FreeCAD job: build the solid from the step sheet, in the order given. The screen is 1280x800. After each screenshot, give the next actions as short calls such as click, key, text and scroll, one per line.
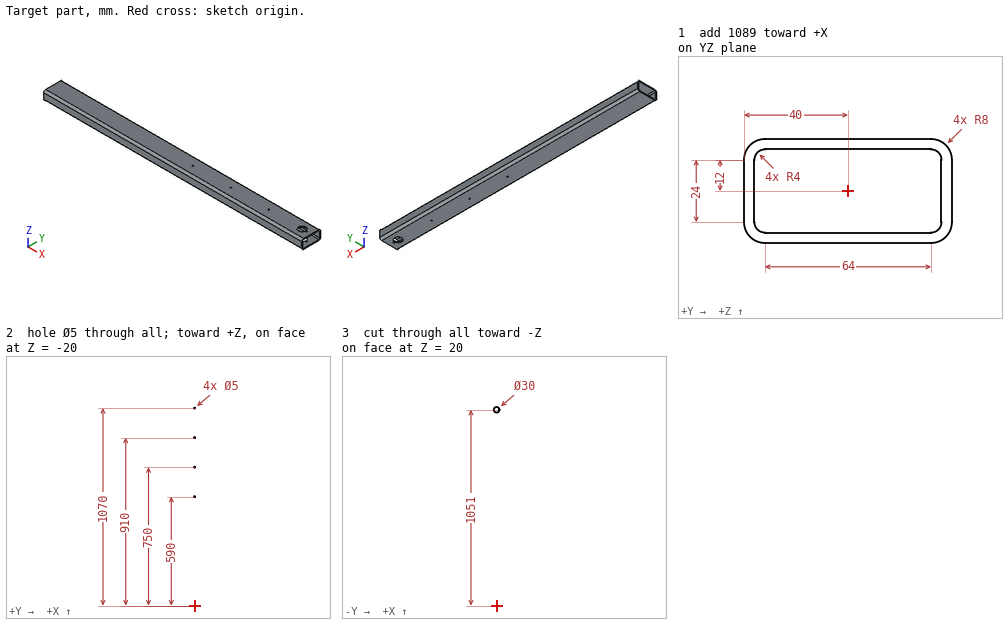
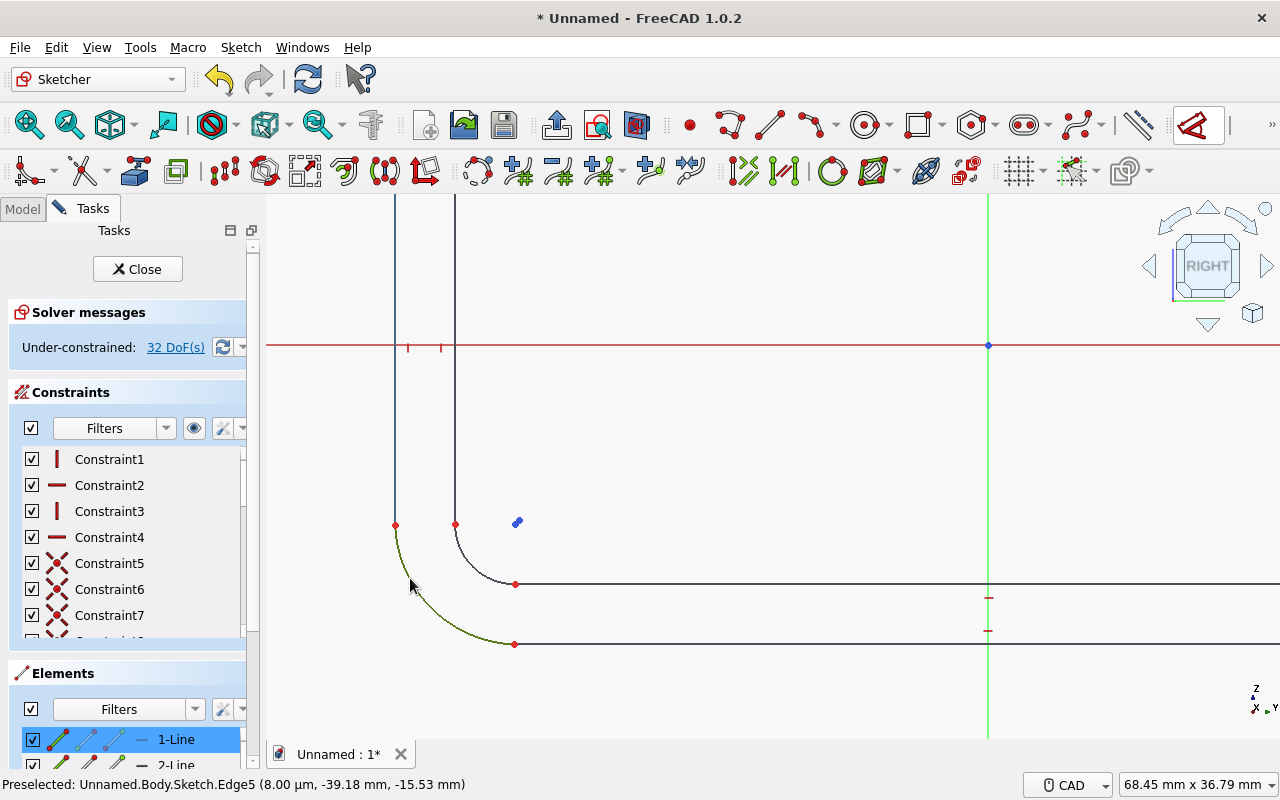
key(t)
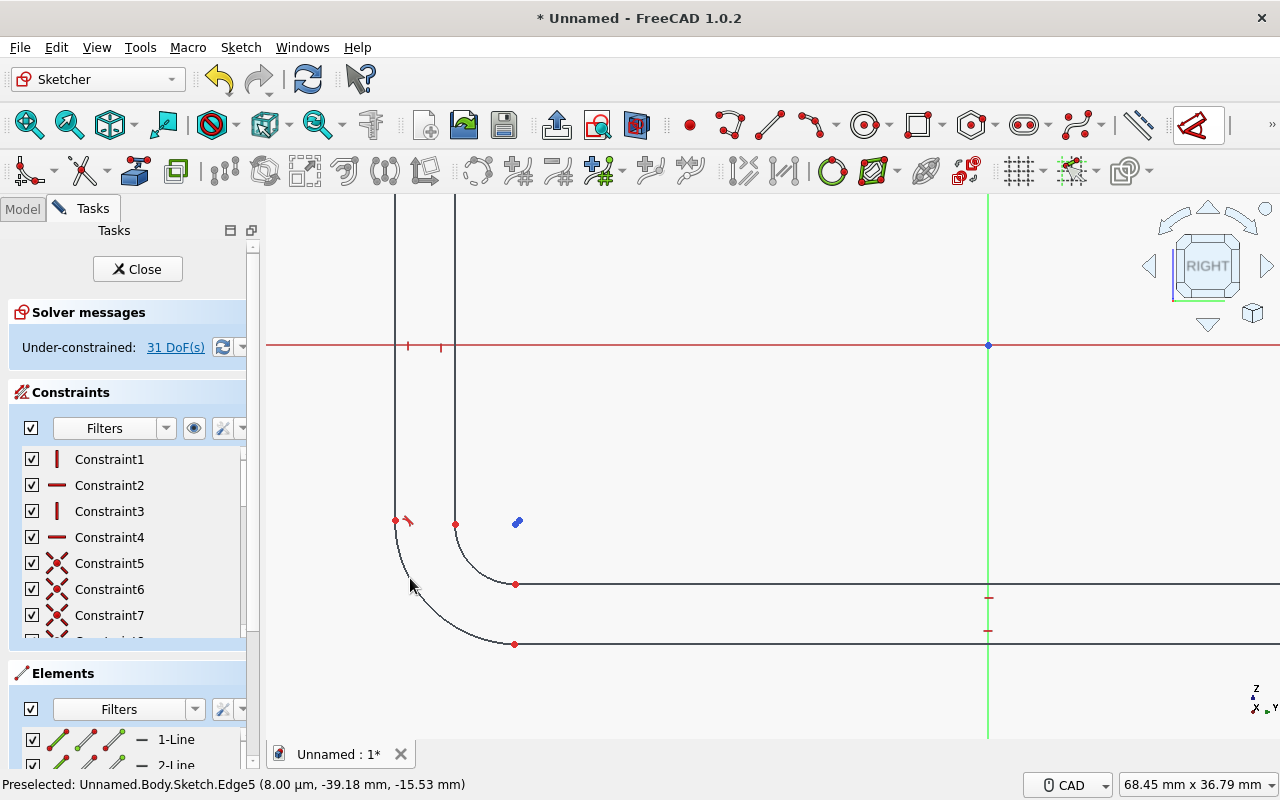
click(395, 275)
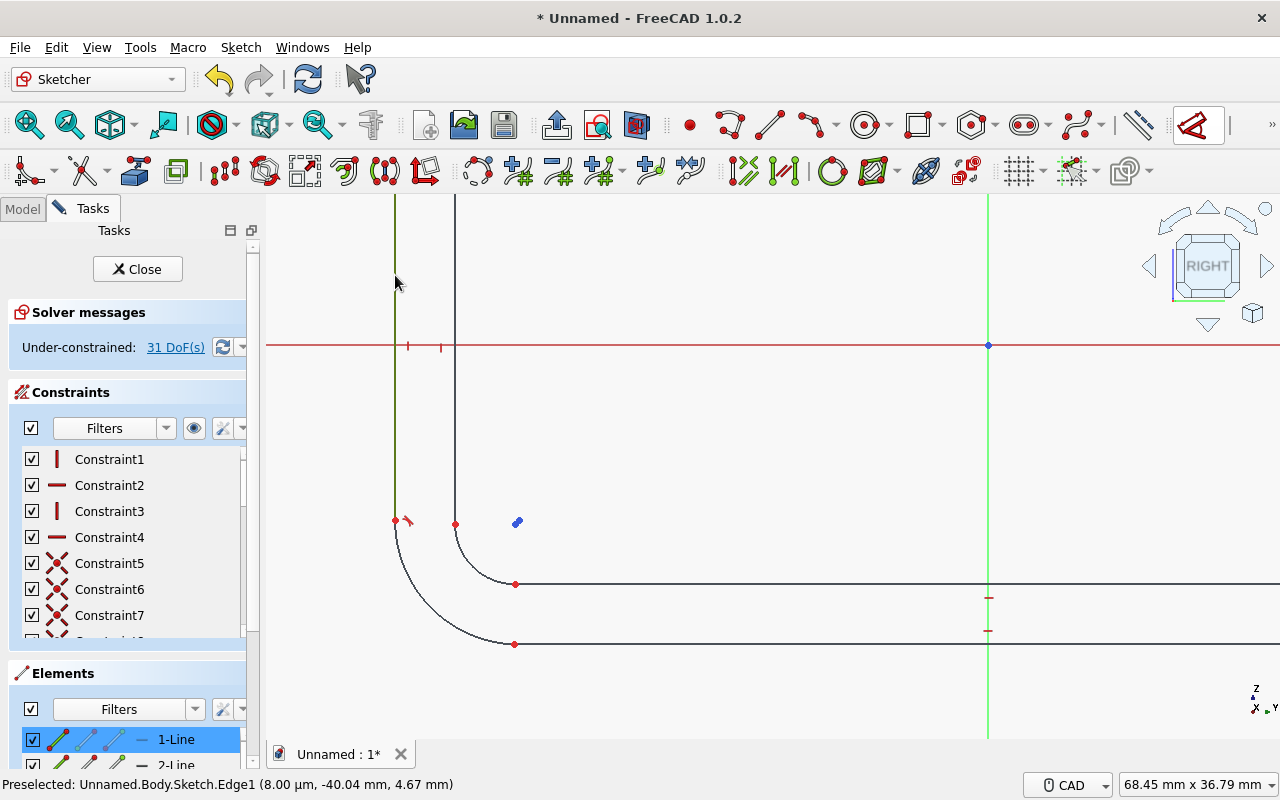
scroll(473, 566, down, 4)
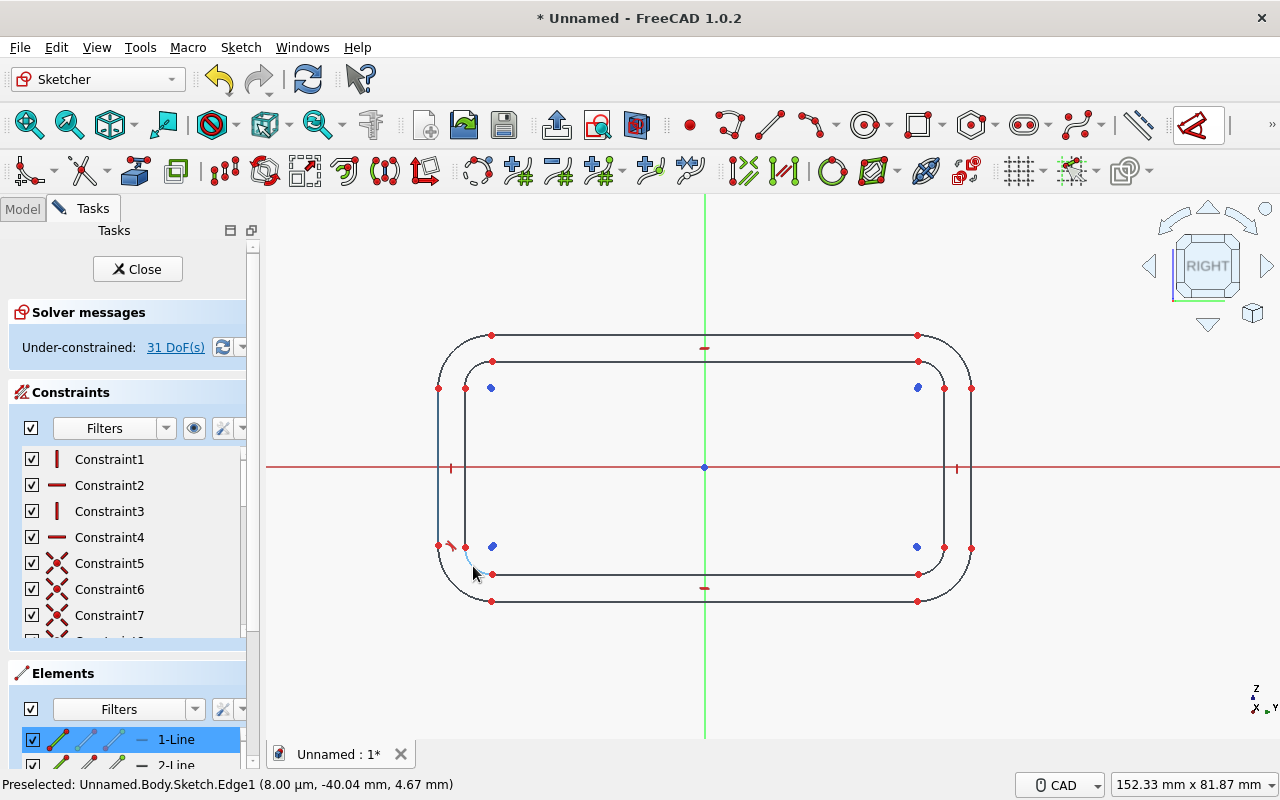
click(467, 341)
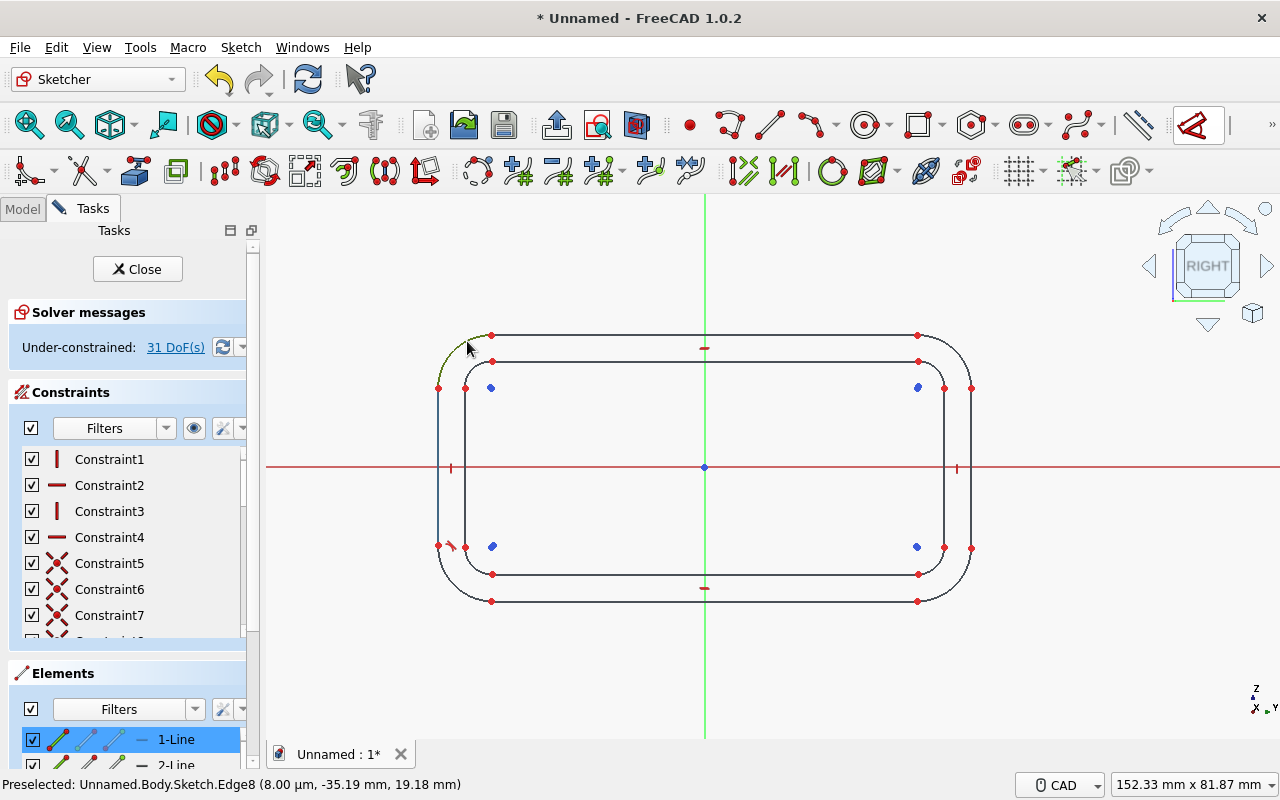
key(t)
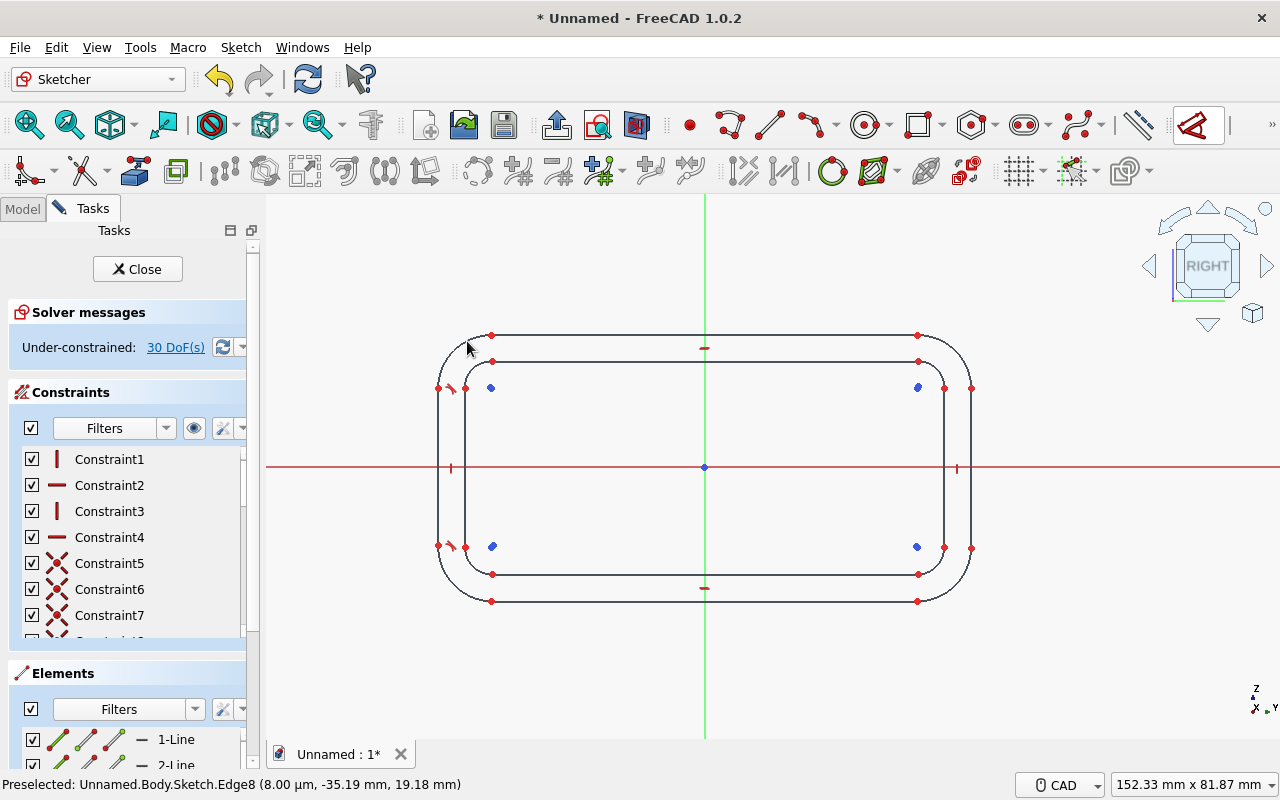
click(619, 602)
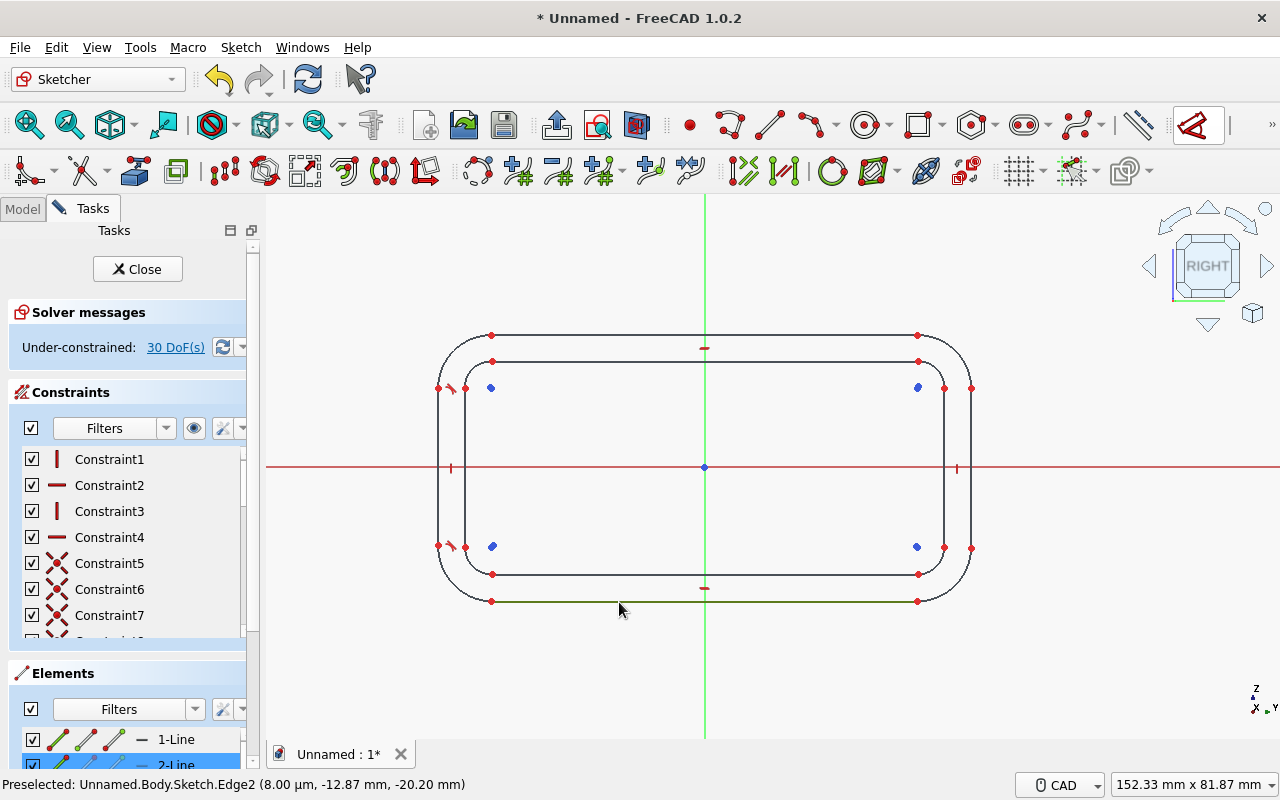
click(444, 571)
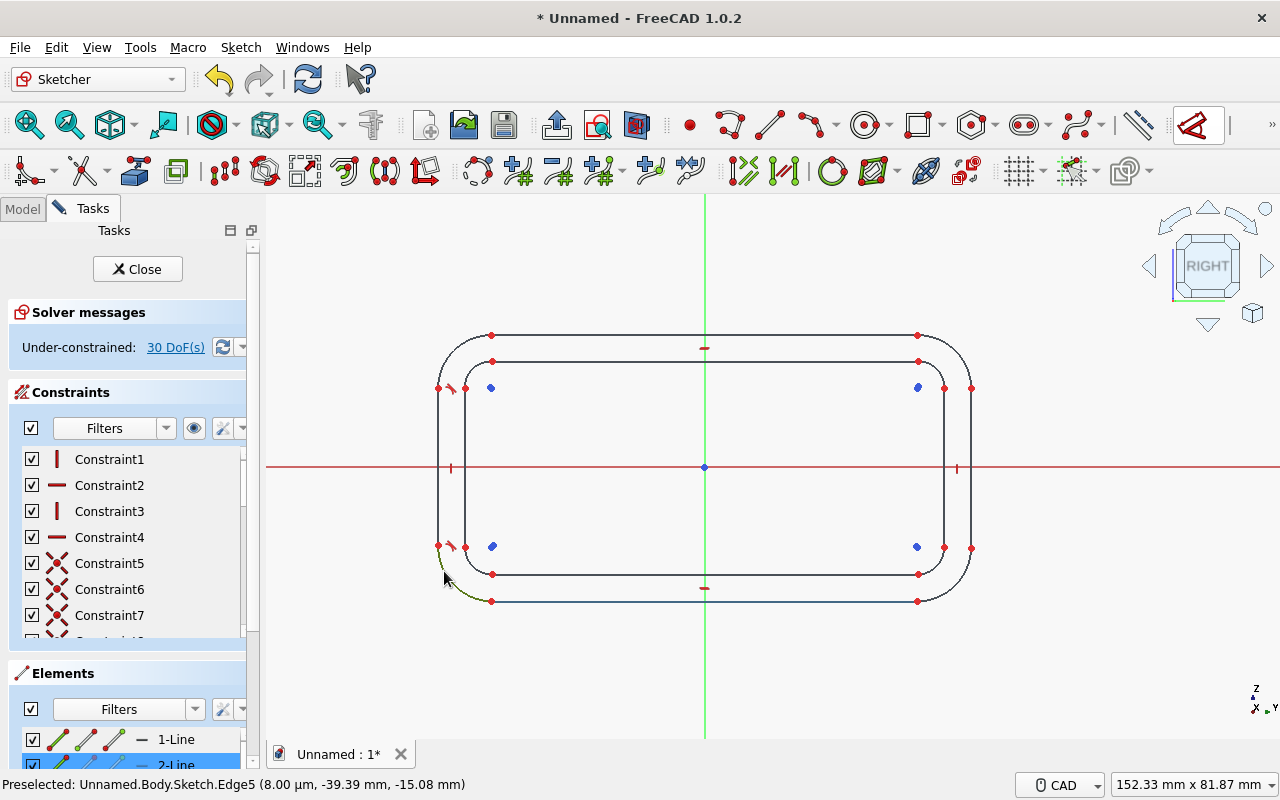
key(t)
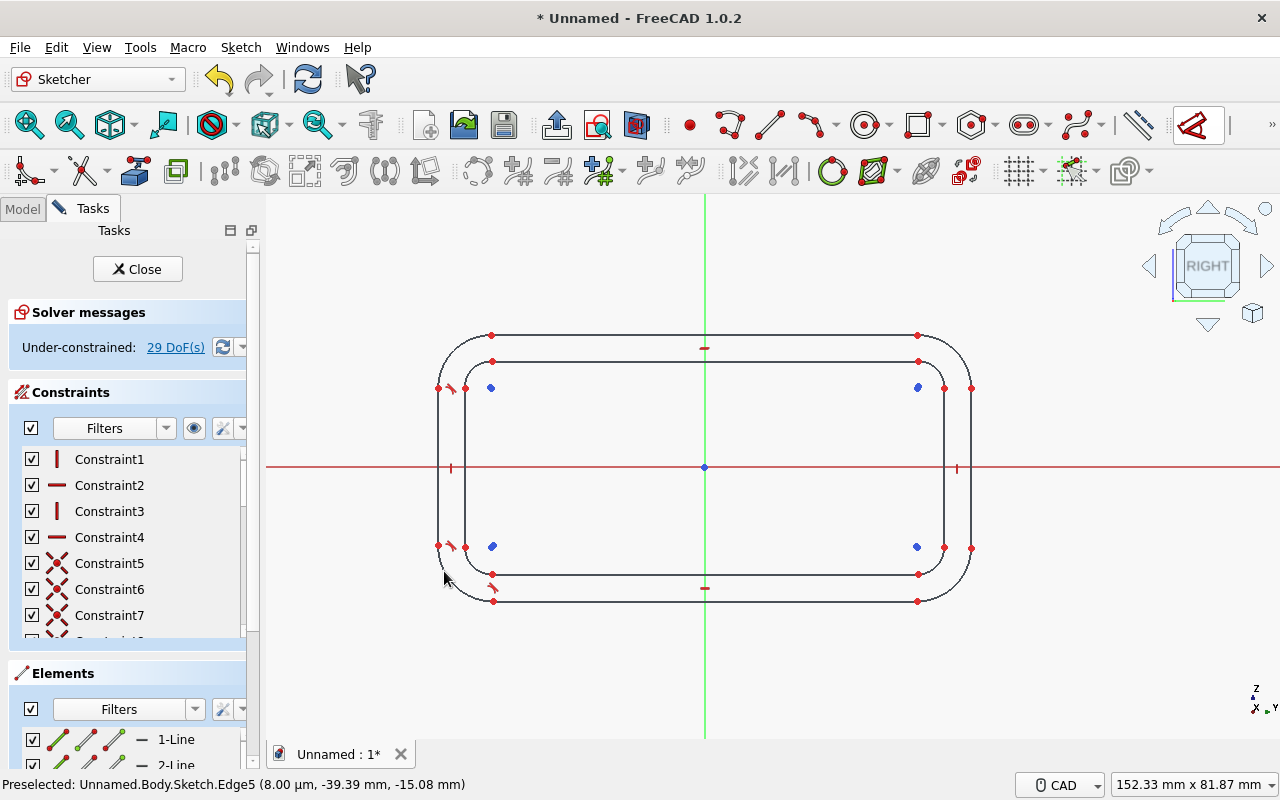
click(621, 602)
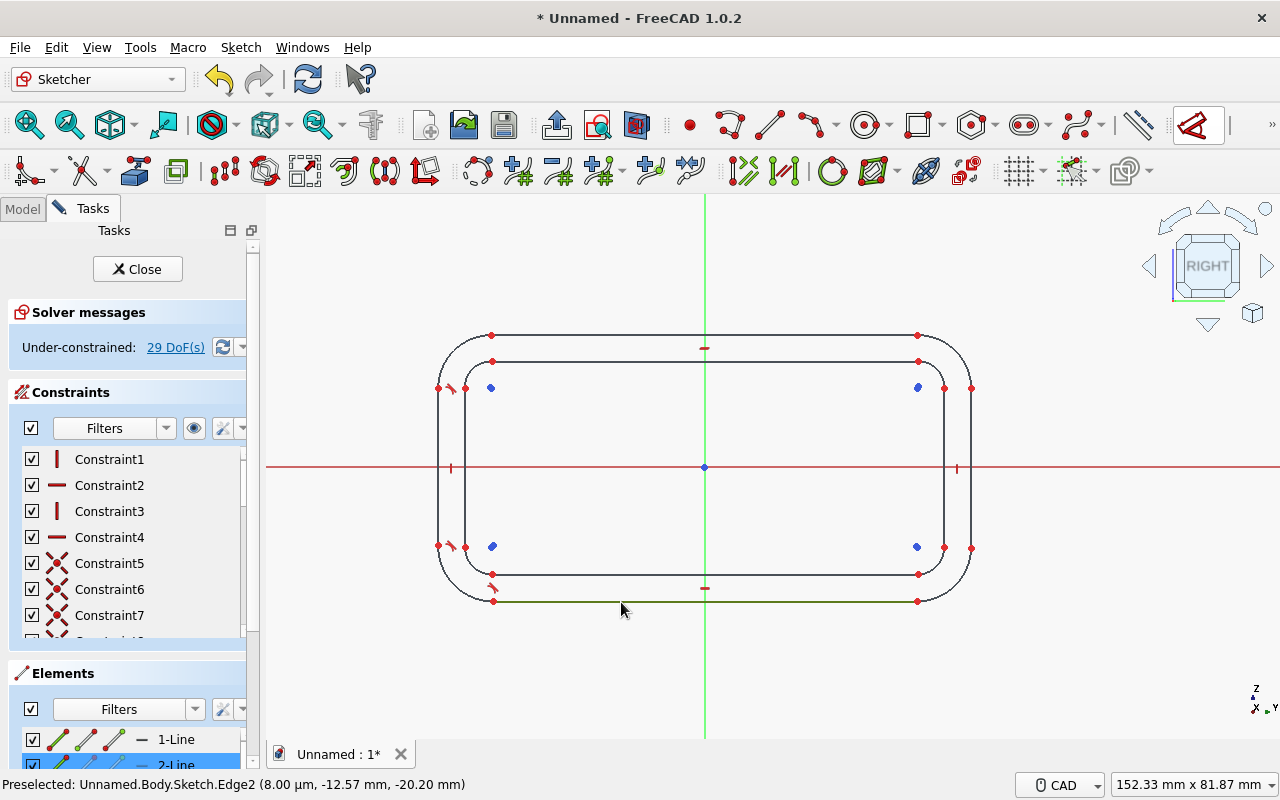
click(942, 595)